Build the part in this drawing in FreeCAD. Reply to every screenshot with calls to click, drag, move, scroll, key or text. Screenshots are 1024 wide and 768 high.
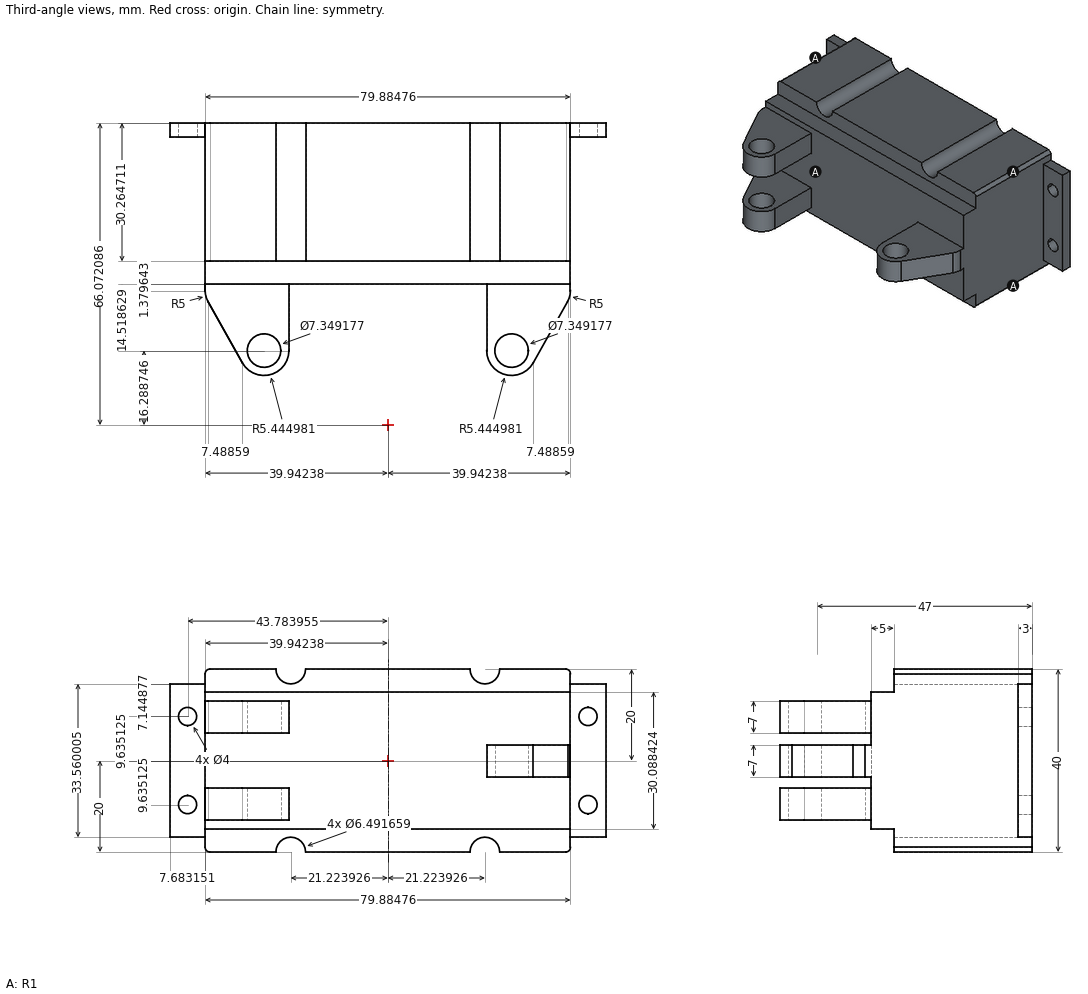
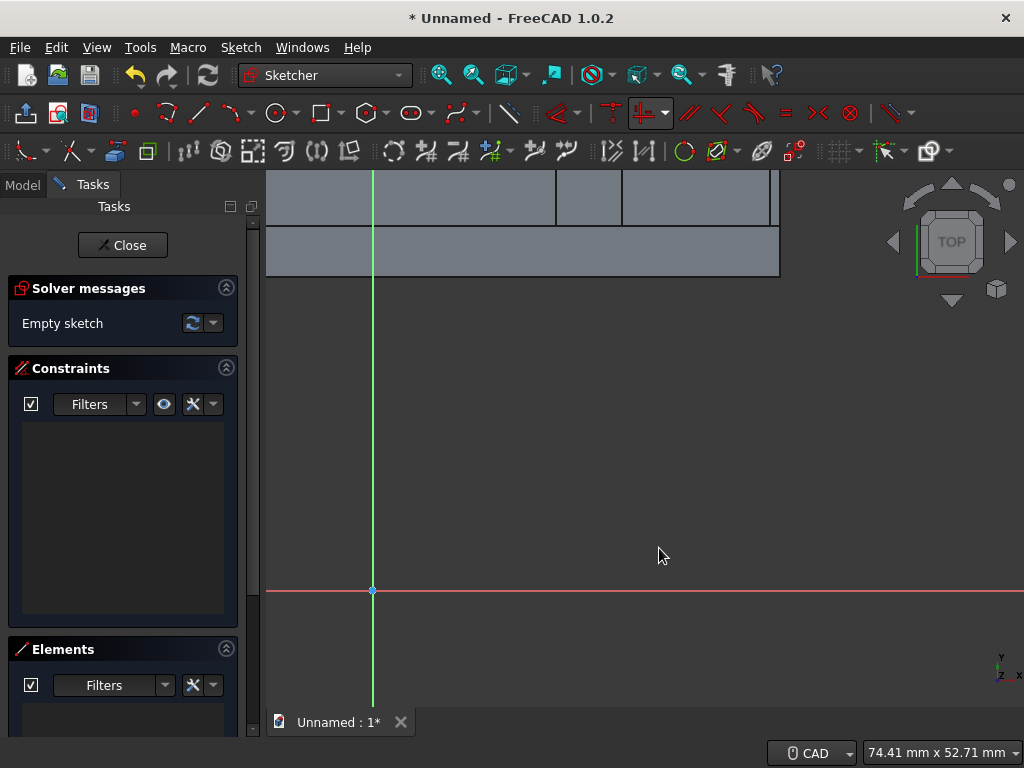
click(200, 114)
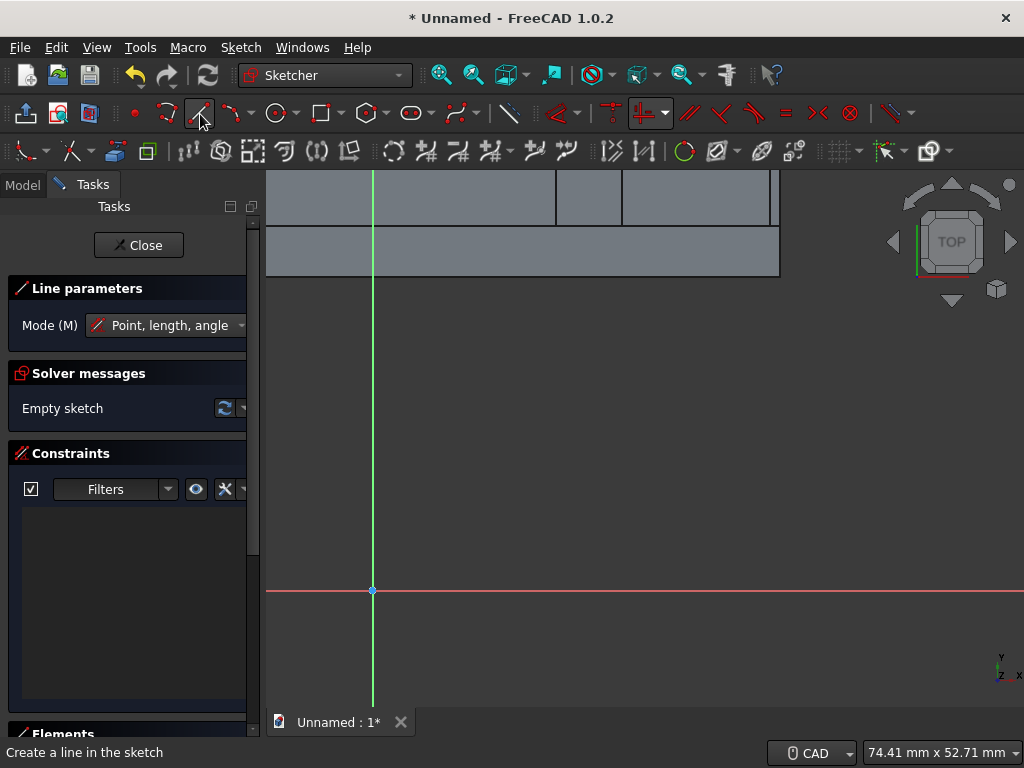
click(697, 452)
click(773, 316)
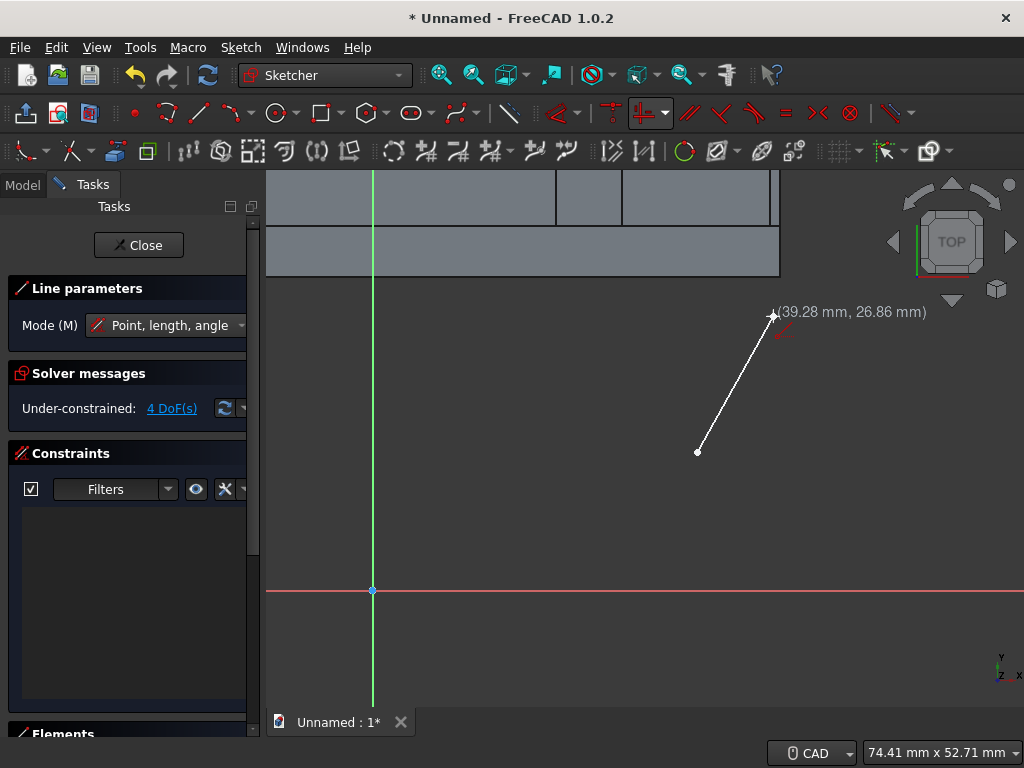
click(168, 114)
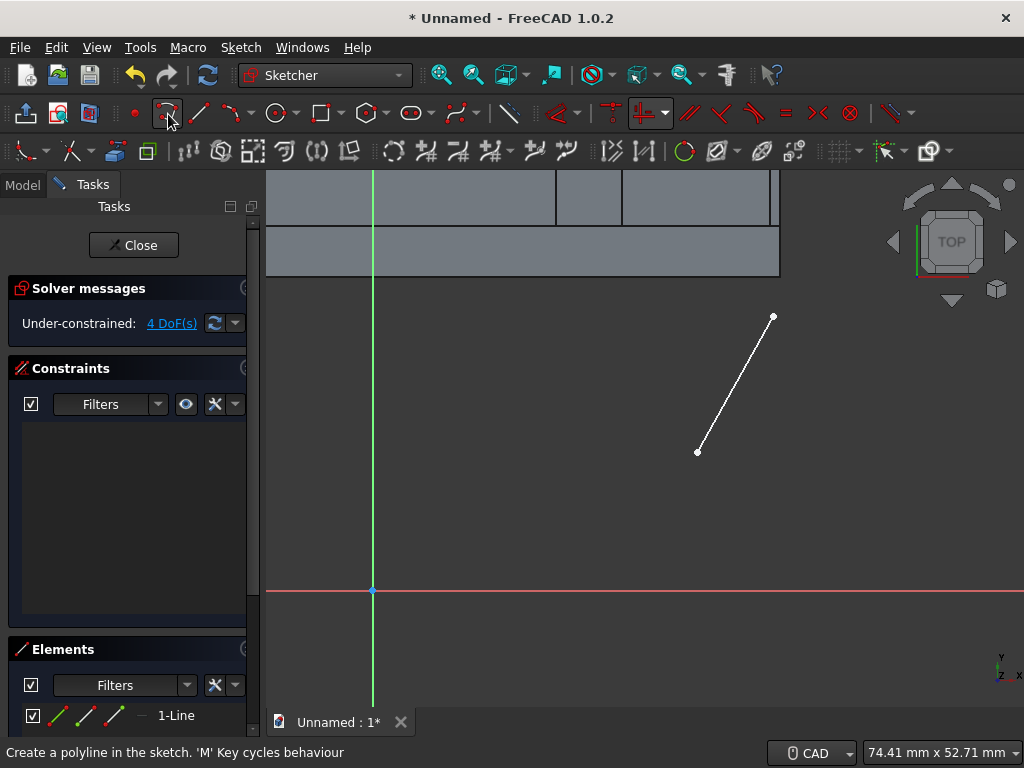
click(780, 291)
click(780, 277)
click(593, 277)
click(593, 425)
right_click(593, 425)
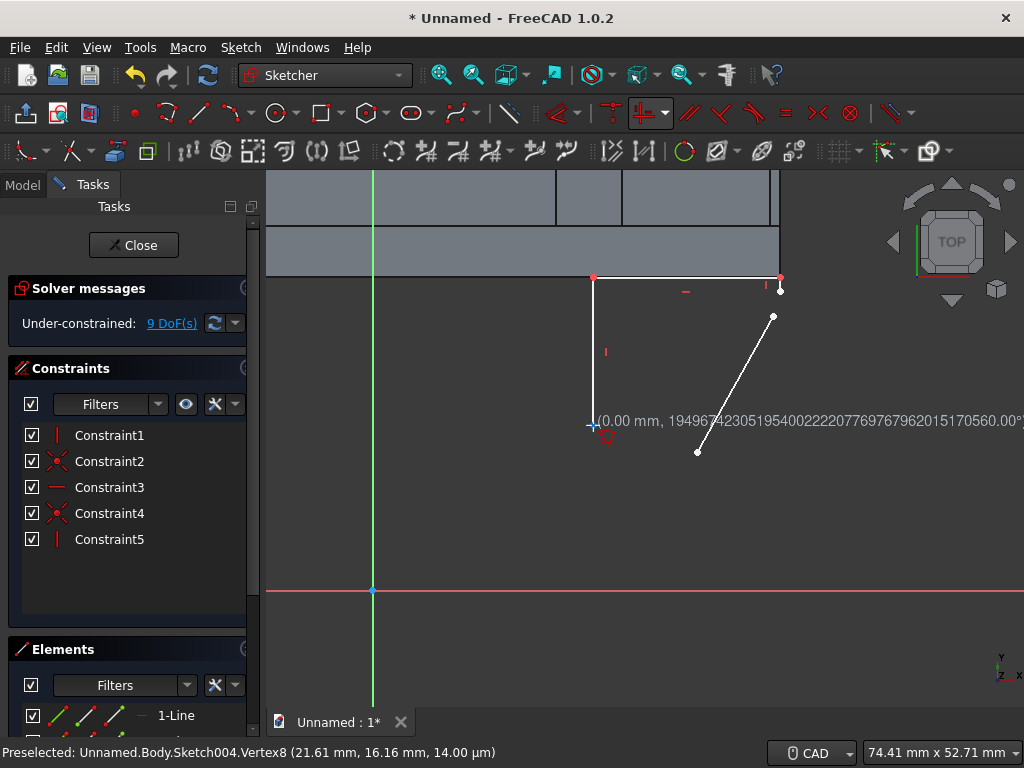
click(232, 114)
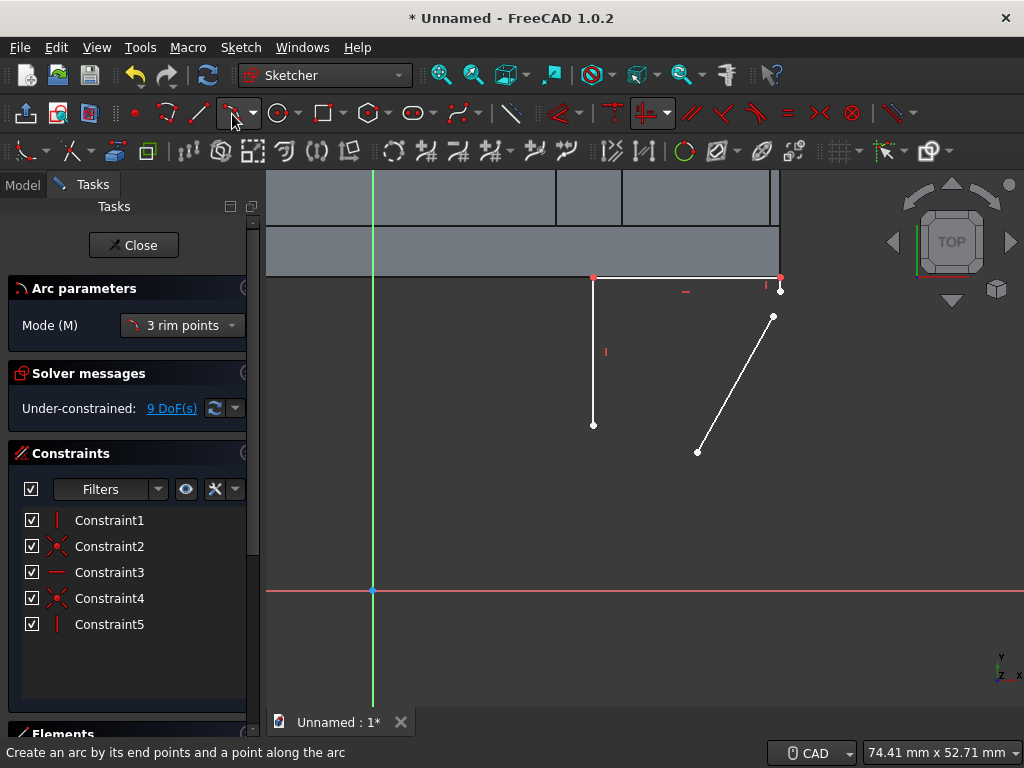
click(773, 317)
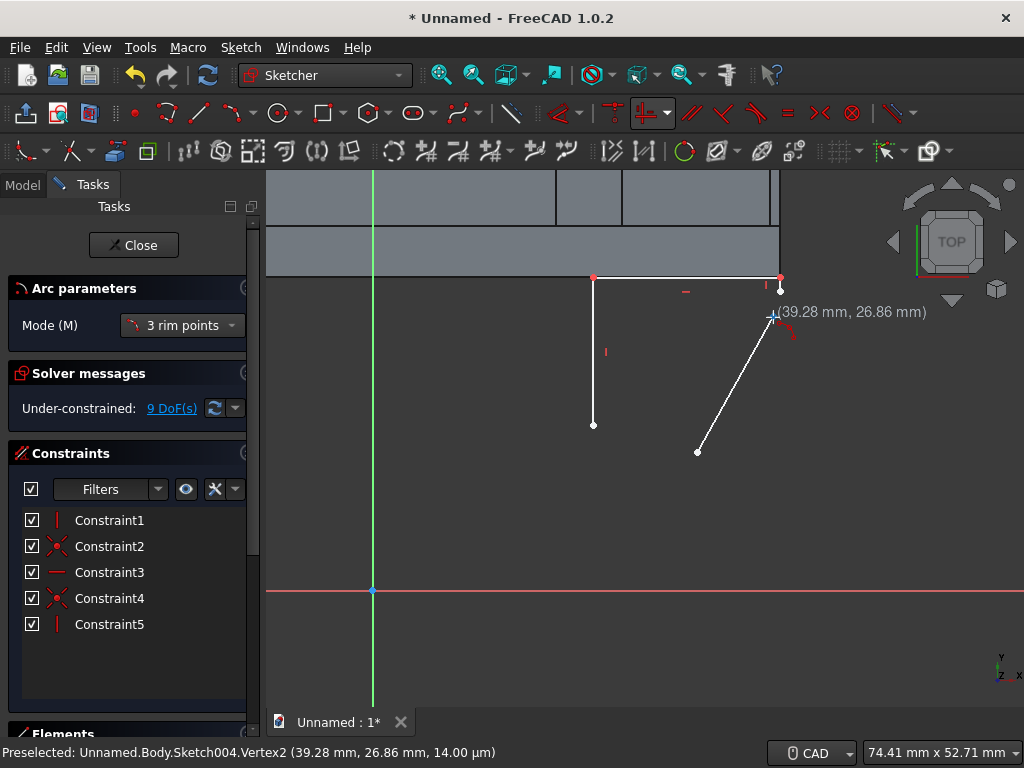
scroll(780, 291, up, 5)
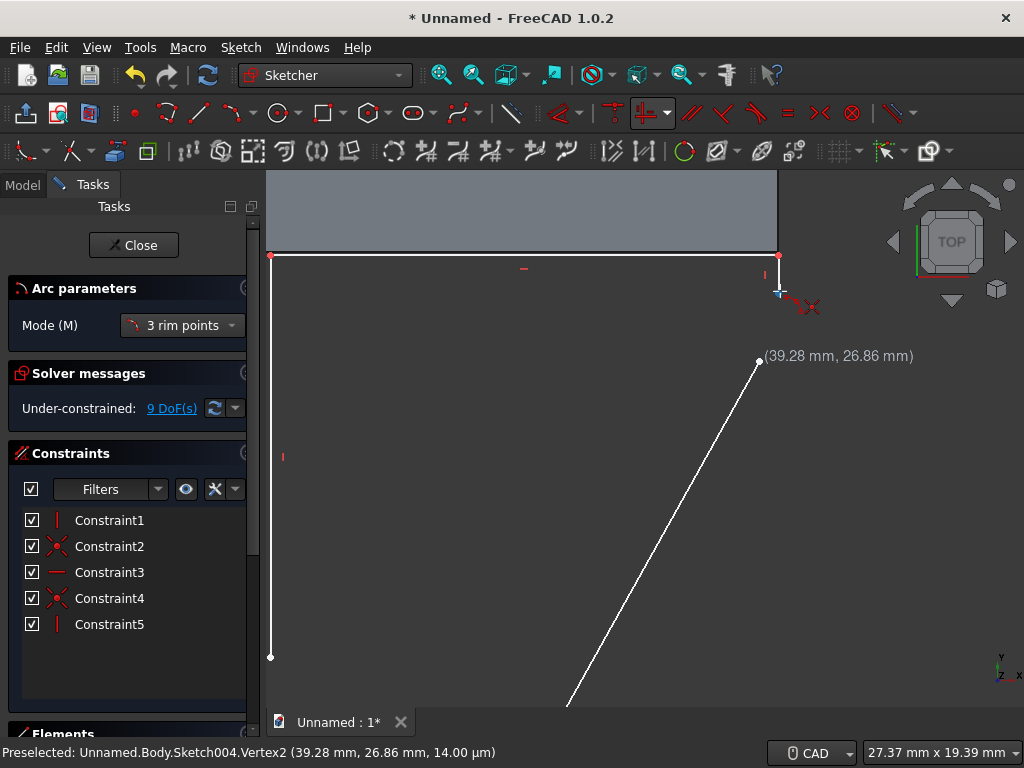
click(779, 293)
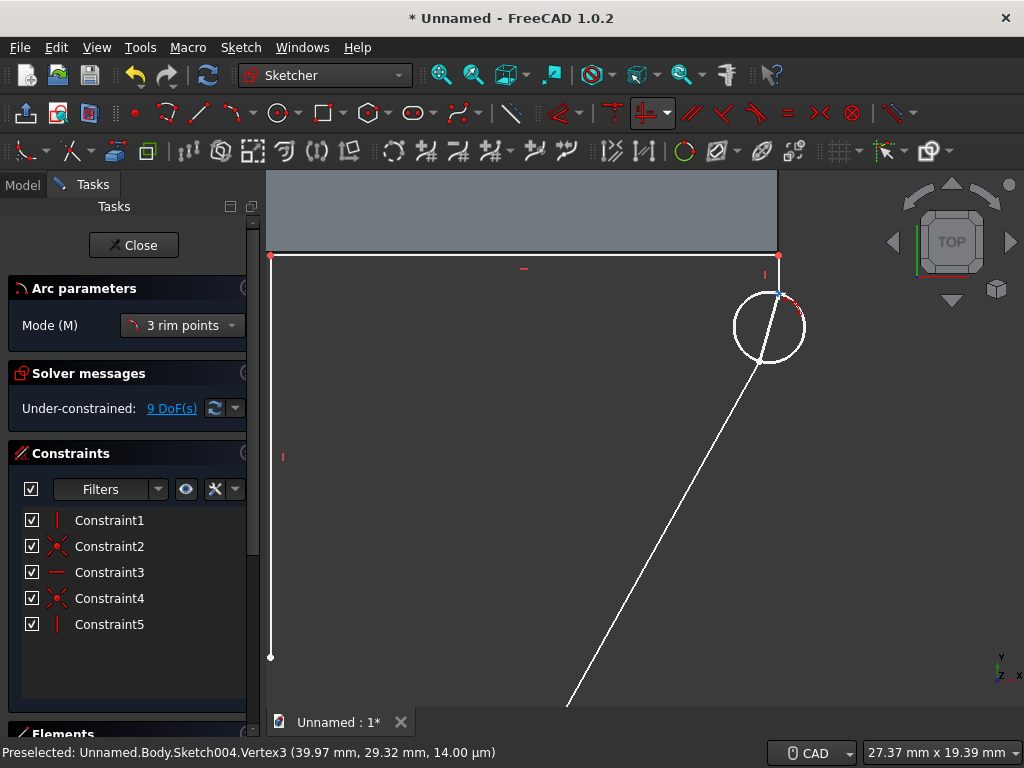
scroll(774, 325, up, 7)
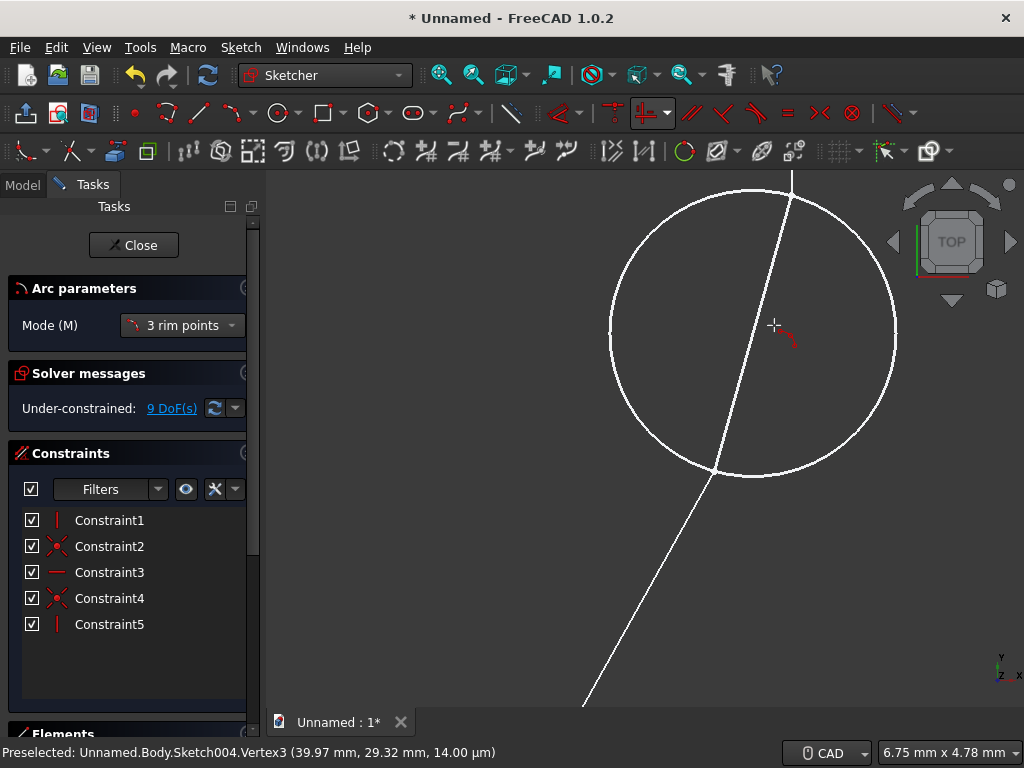
click(771, 325)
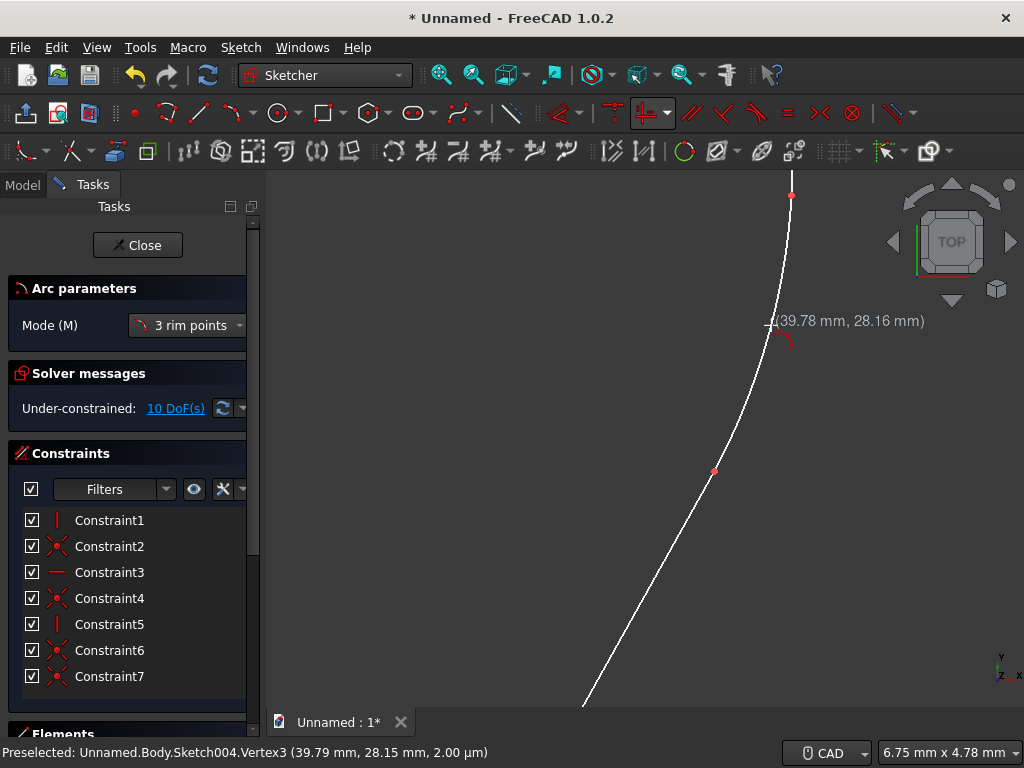
scroll(779, 307, down, 12)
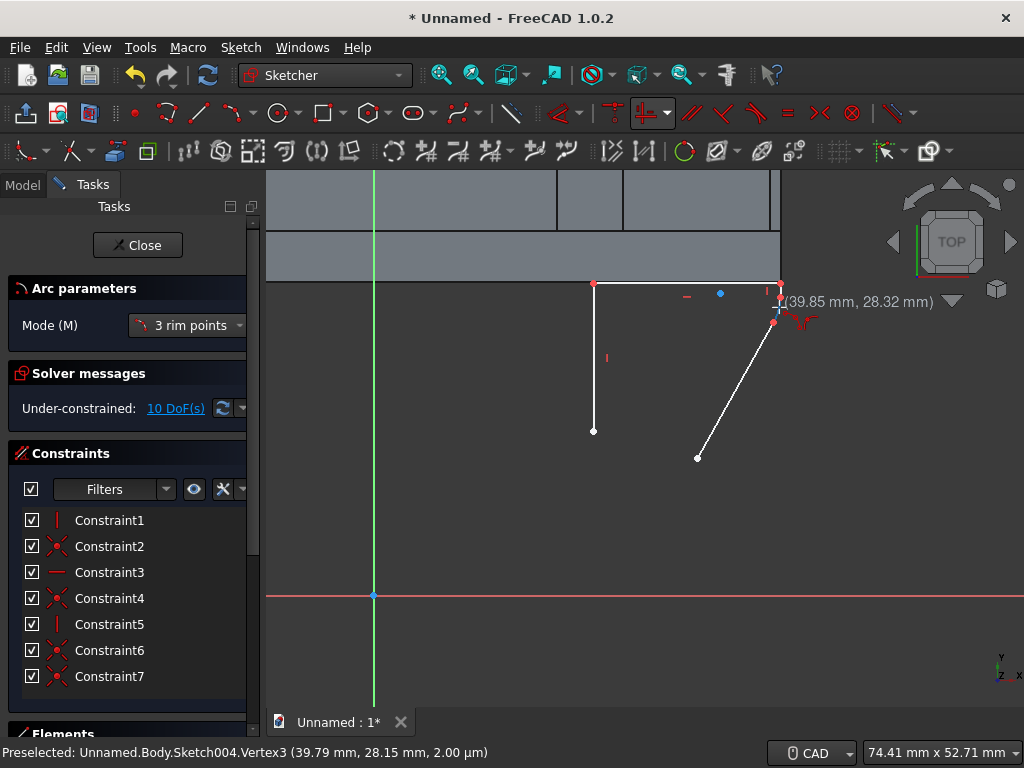
click(594, 431)
click(698, 458)
click(635, 484)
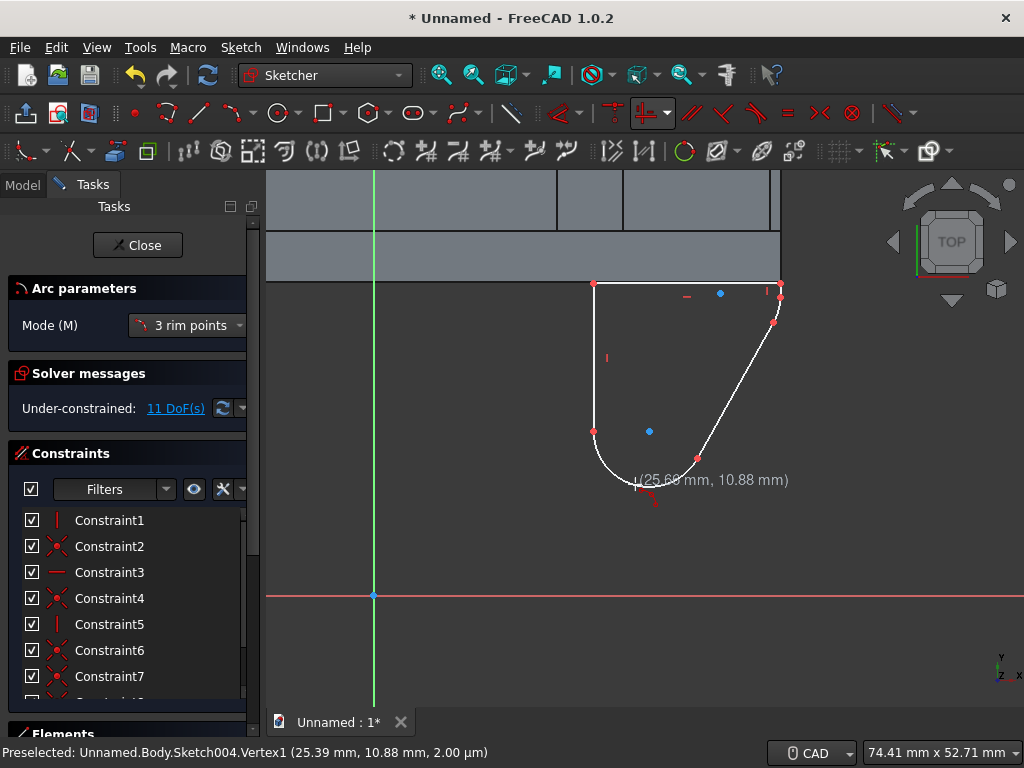
key(g)
key(c)